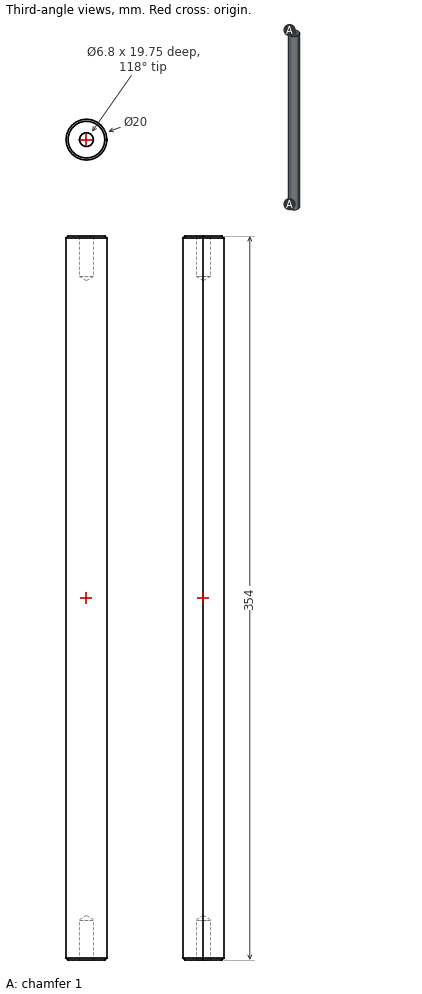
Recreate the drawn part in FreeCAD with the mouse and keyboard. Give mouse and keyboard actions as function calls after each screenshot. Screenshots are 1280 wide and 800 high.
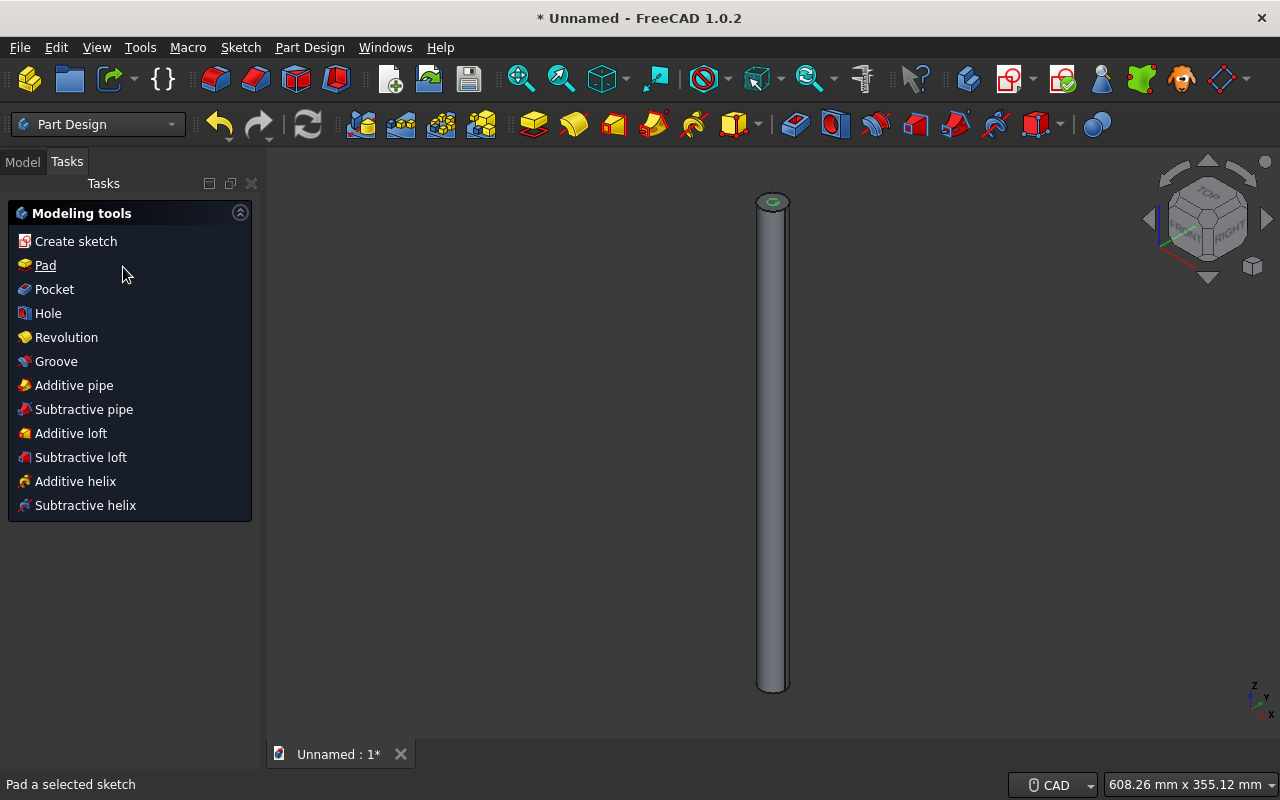
click(836, 124)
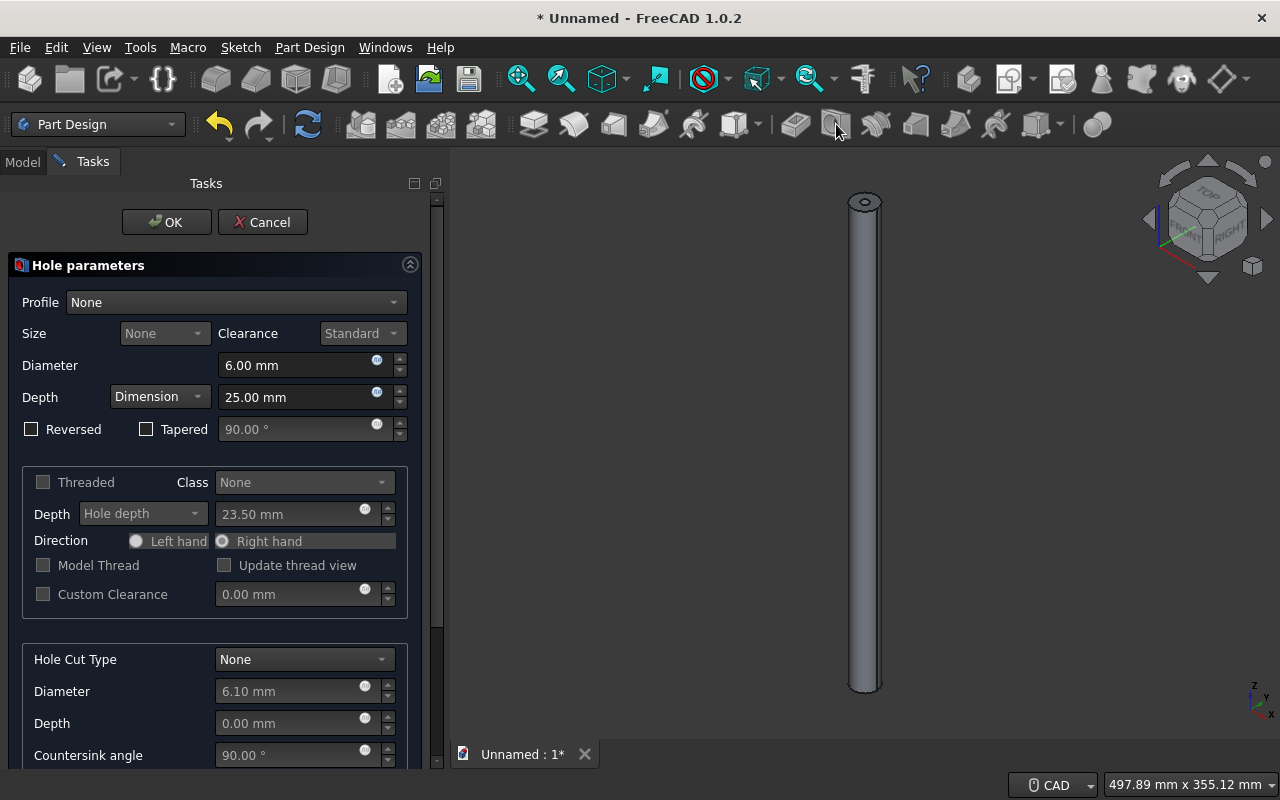
triple_click(305, 365)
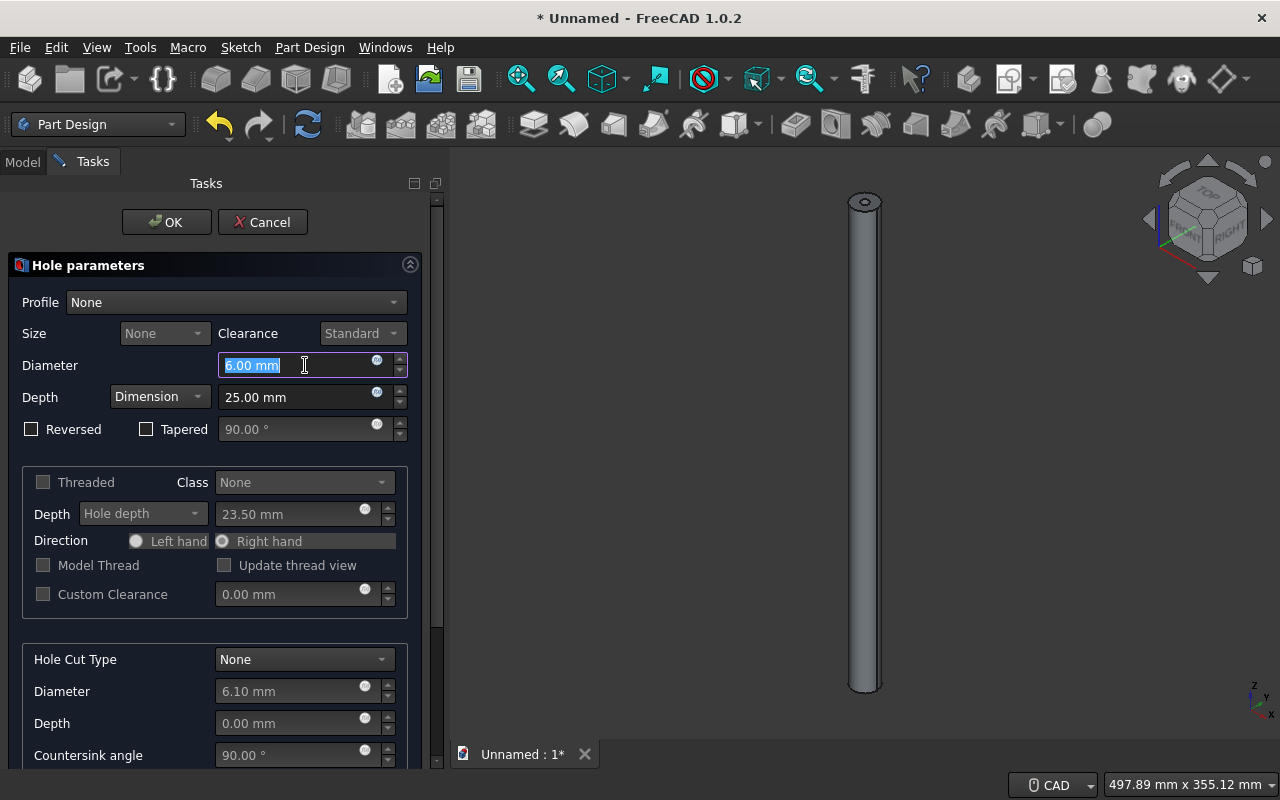
text(6.8)
key(Tab)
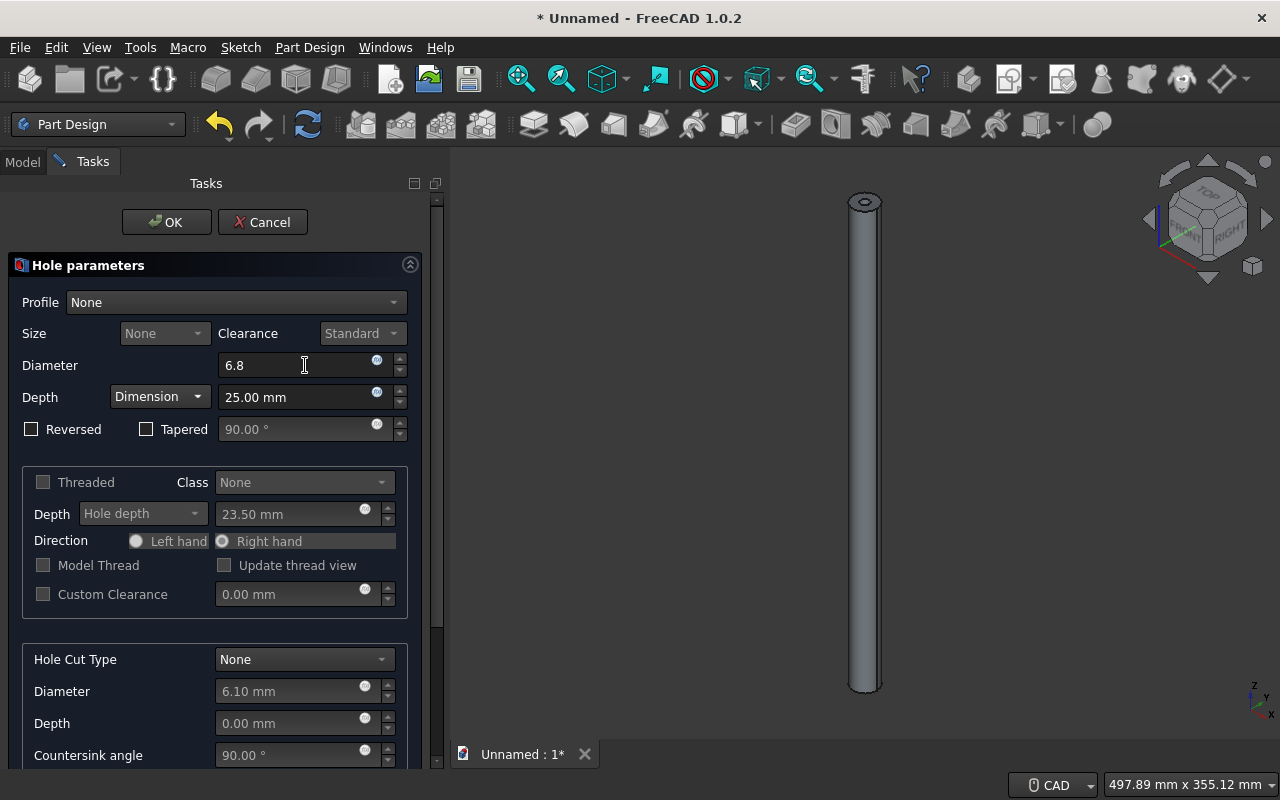
triple_click(305, 397)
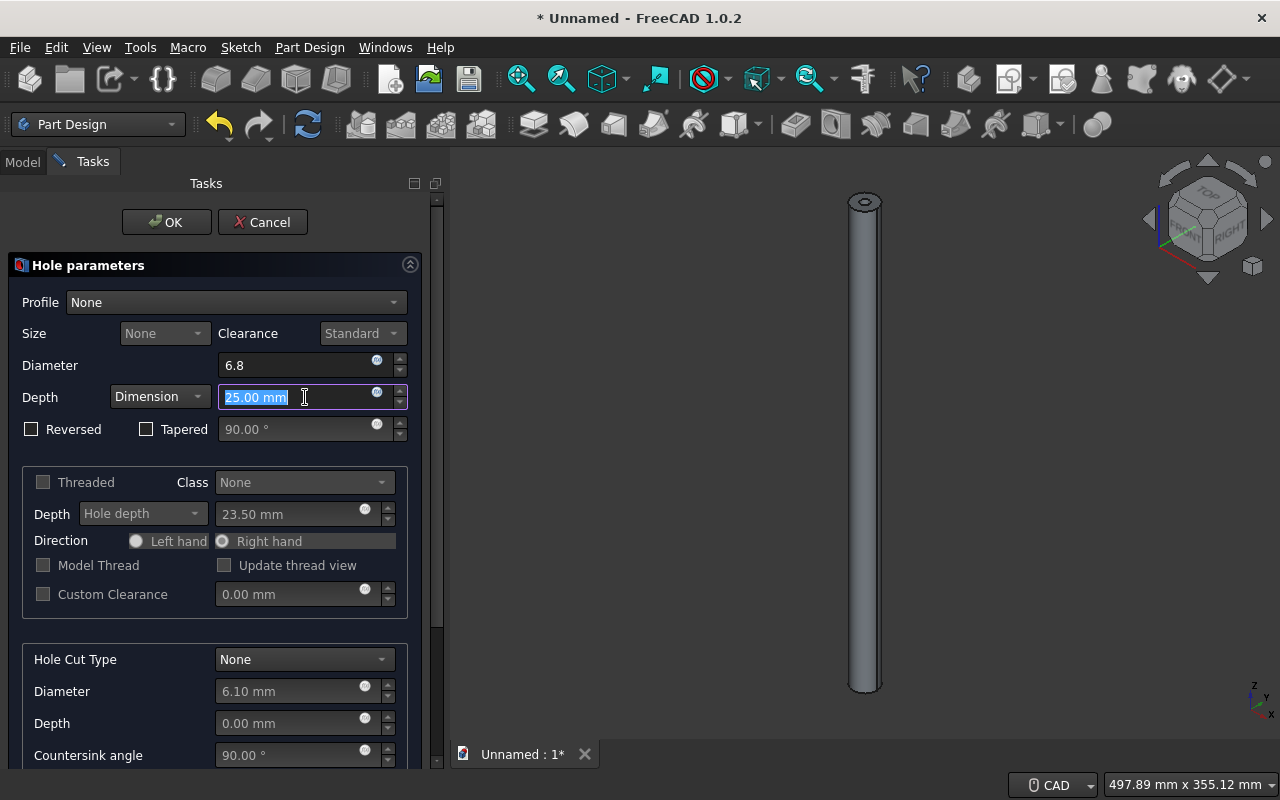
text(19.75)
key(Tab)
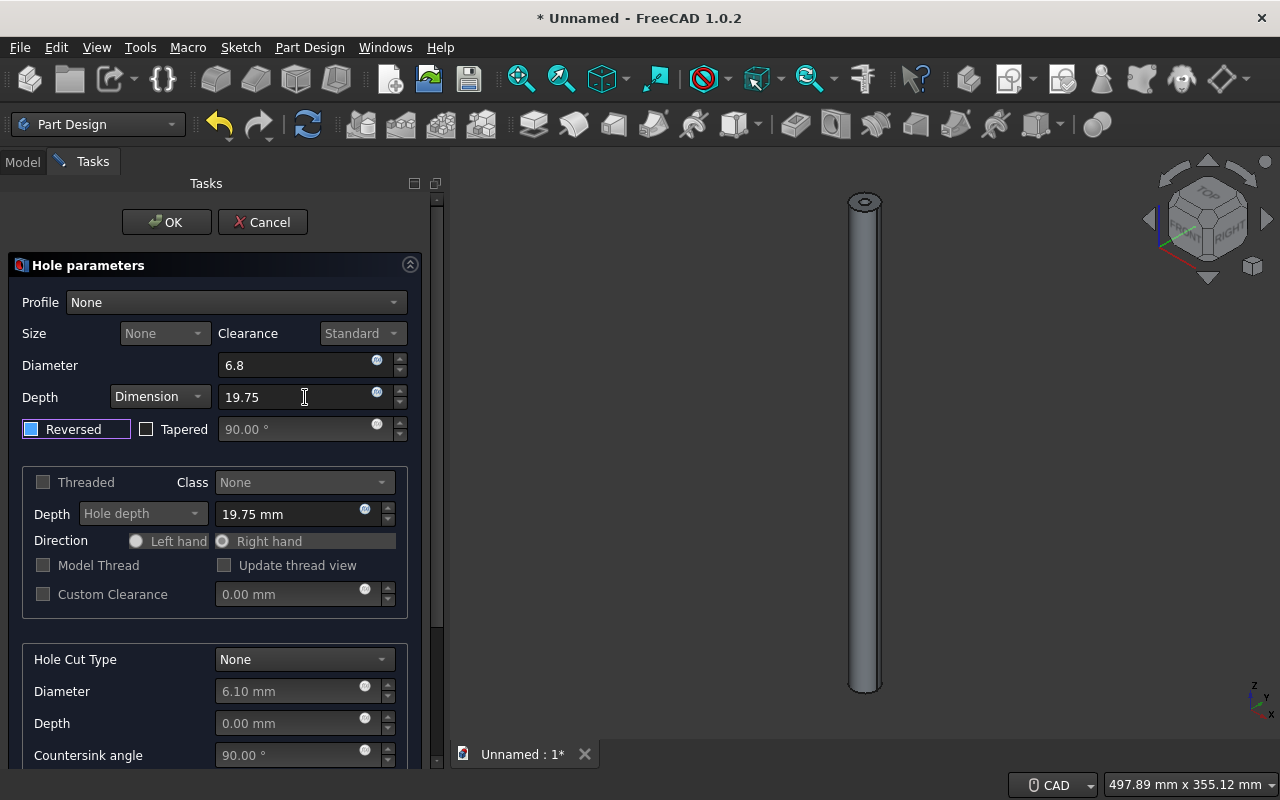
click(167, 222)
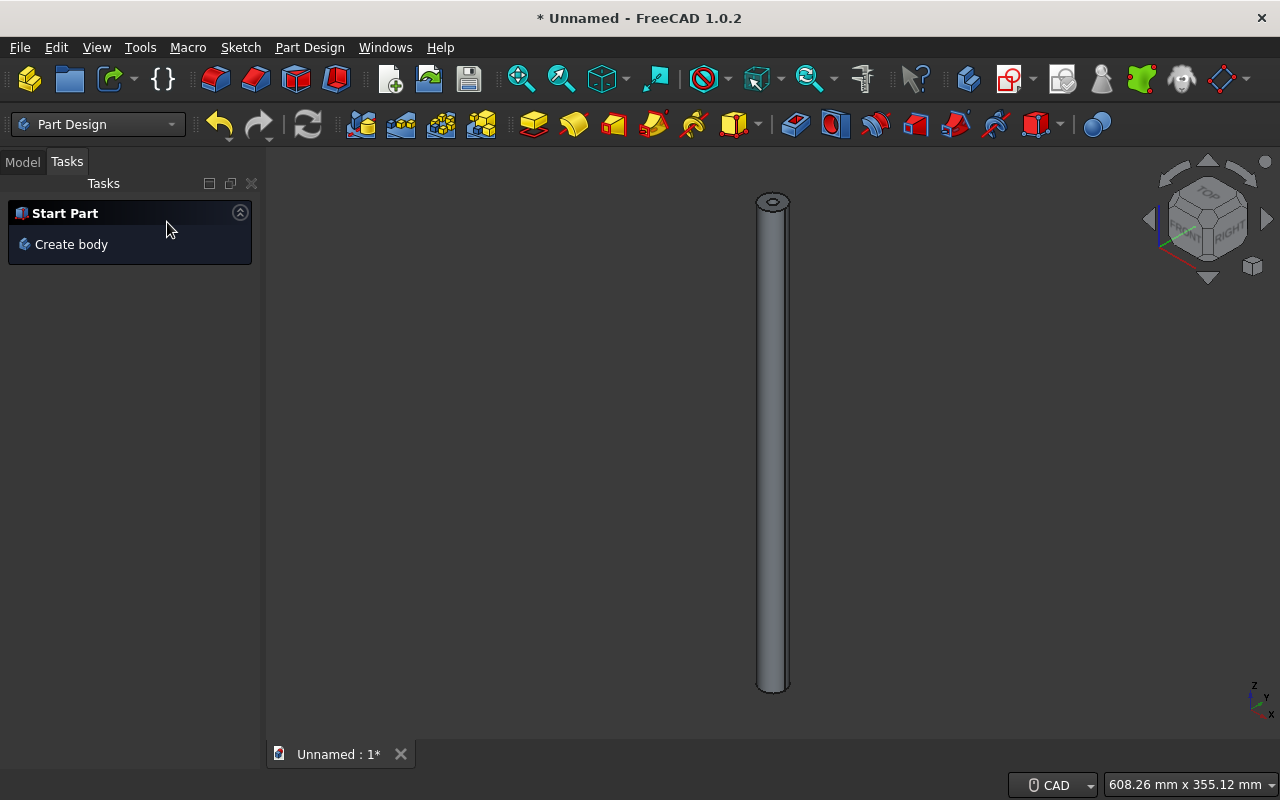
click(761, 194)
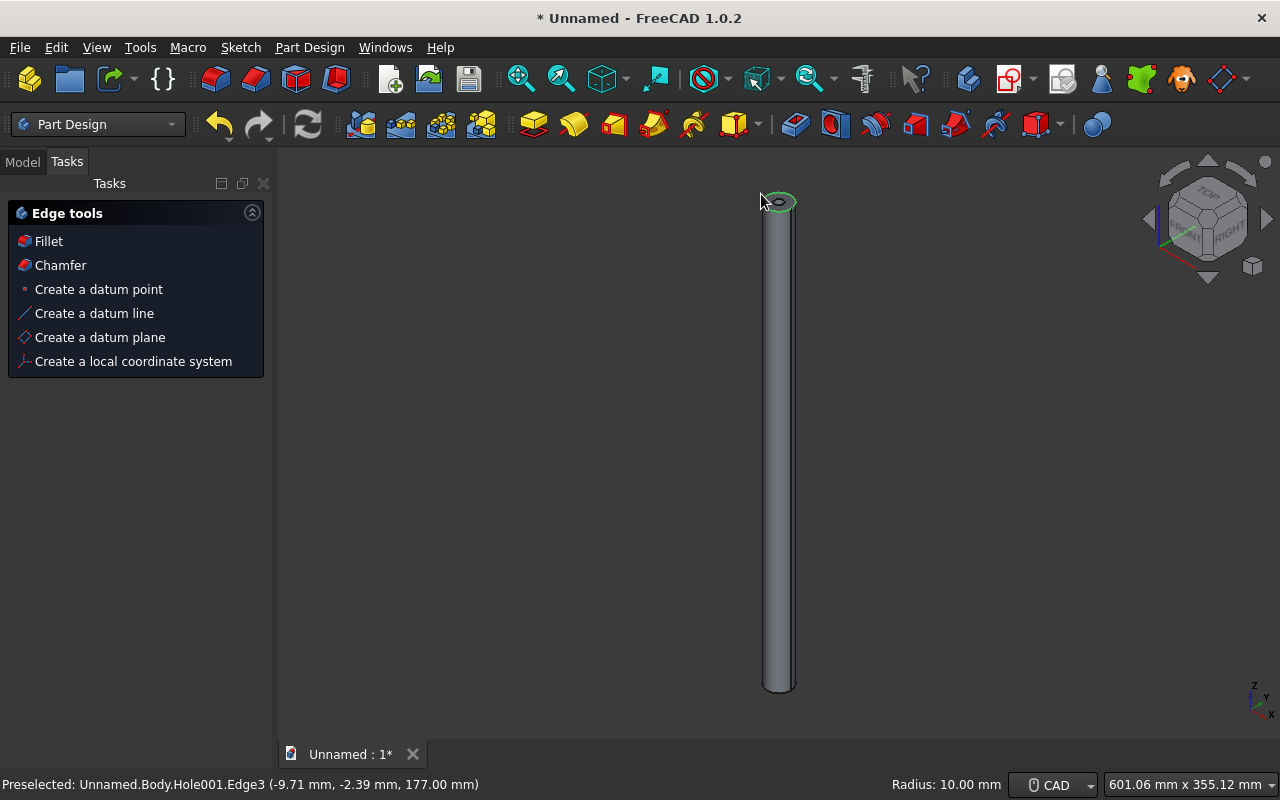
key(2)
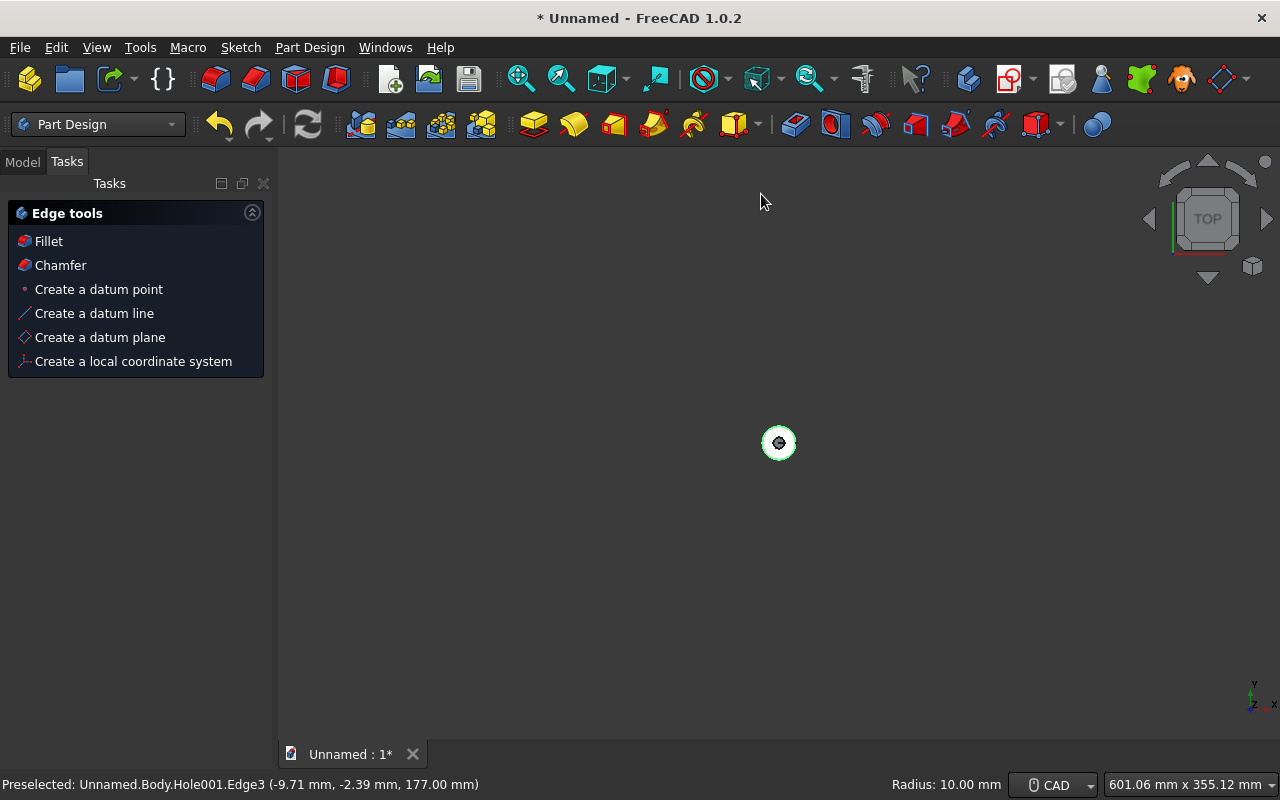
click(522, 80)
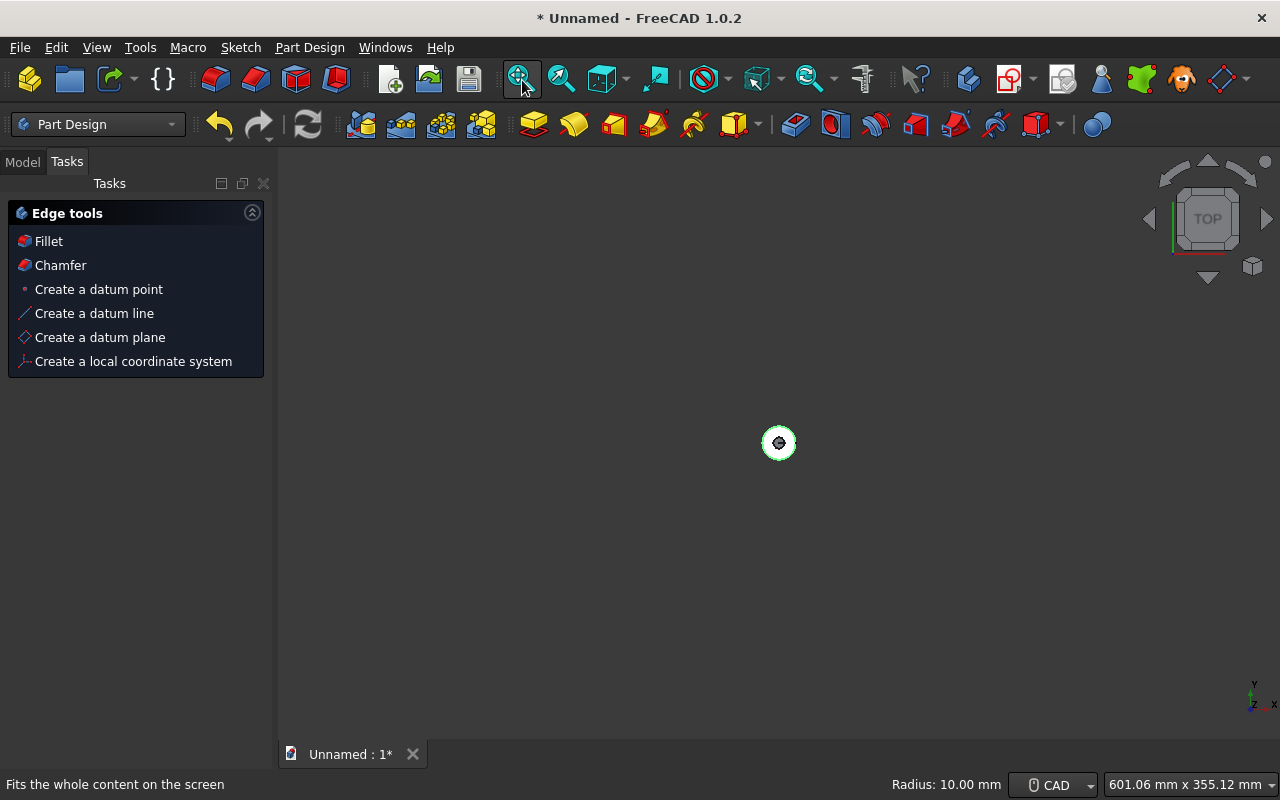
key(0)